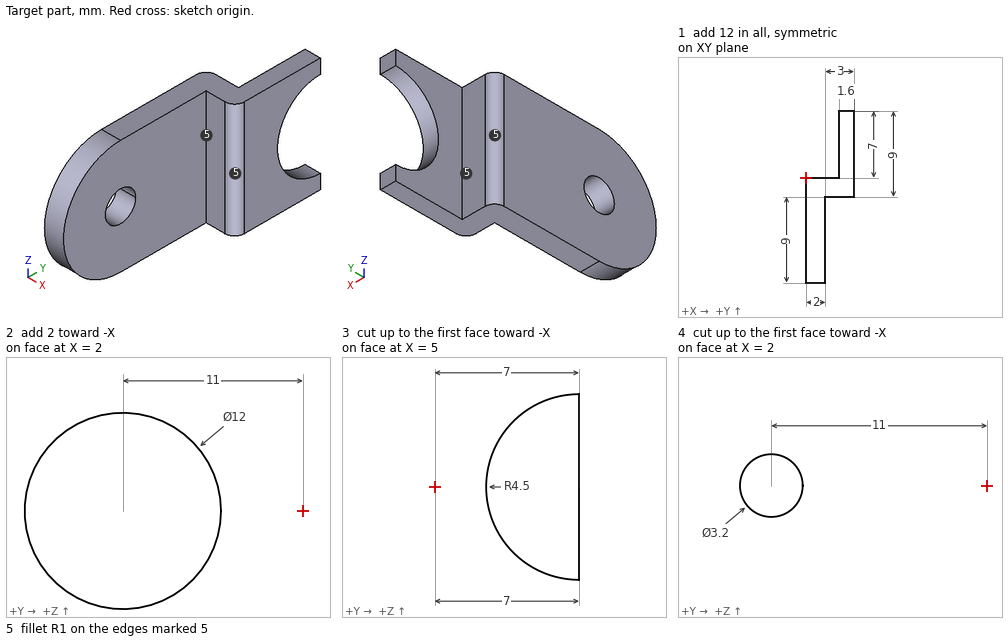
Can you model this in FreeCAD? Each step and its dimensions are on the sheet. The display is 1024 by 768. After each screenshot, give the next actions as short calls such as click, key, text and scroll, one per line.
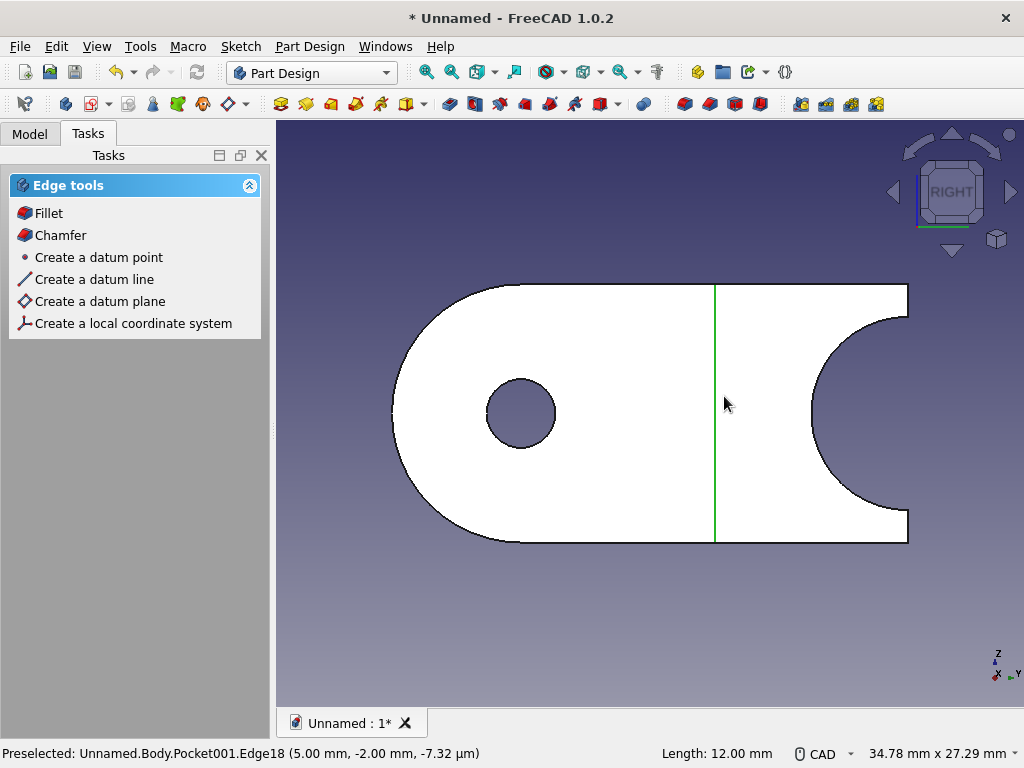
key(5)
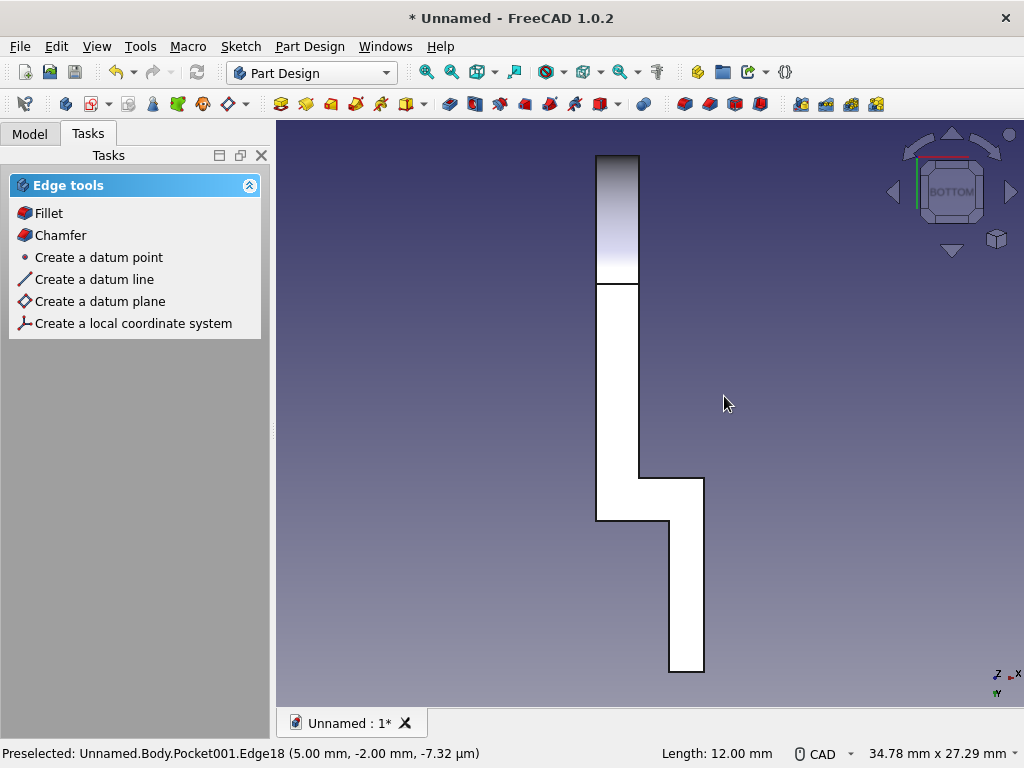
key(4)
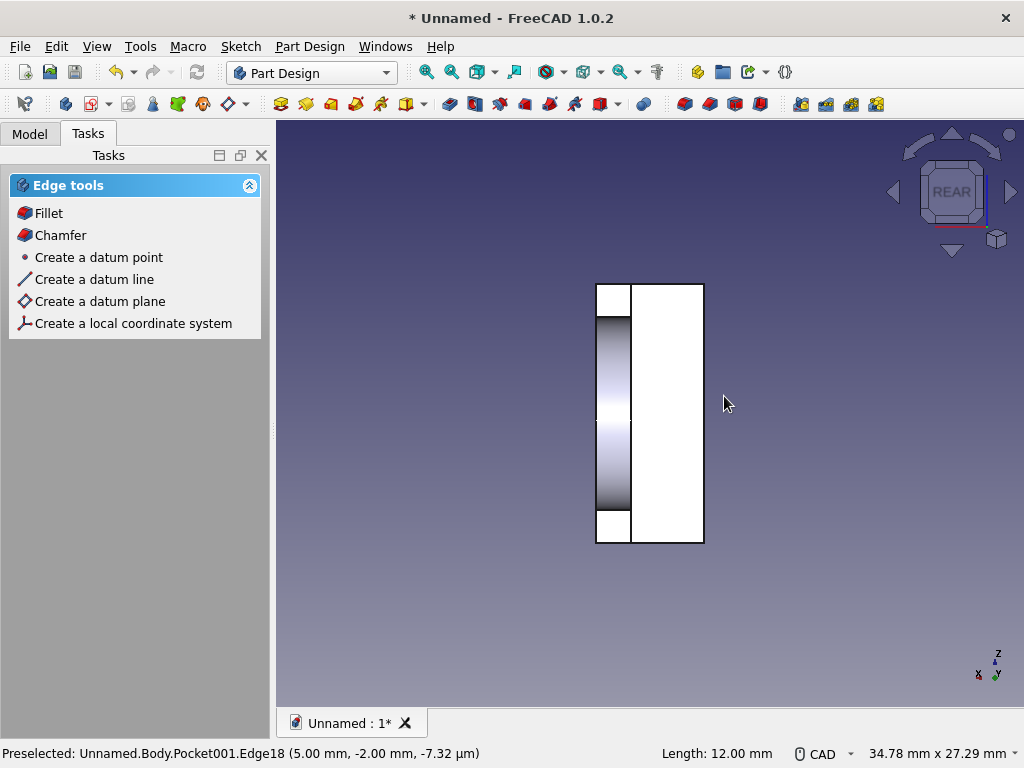
key(v)
key(f)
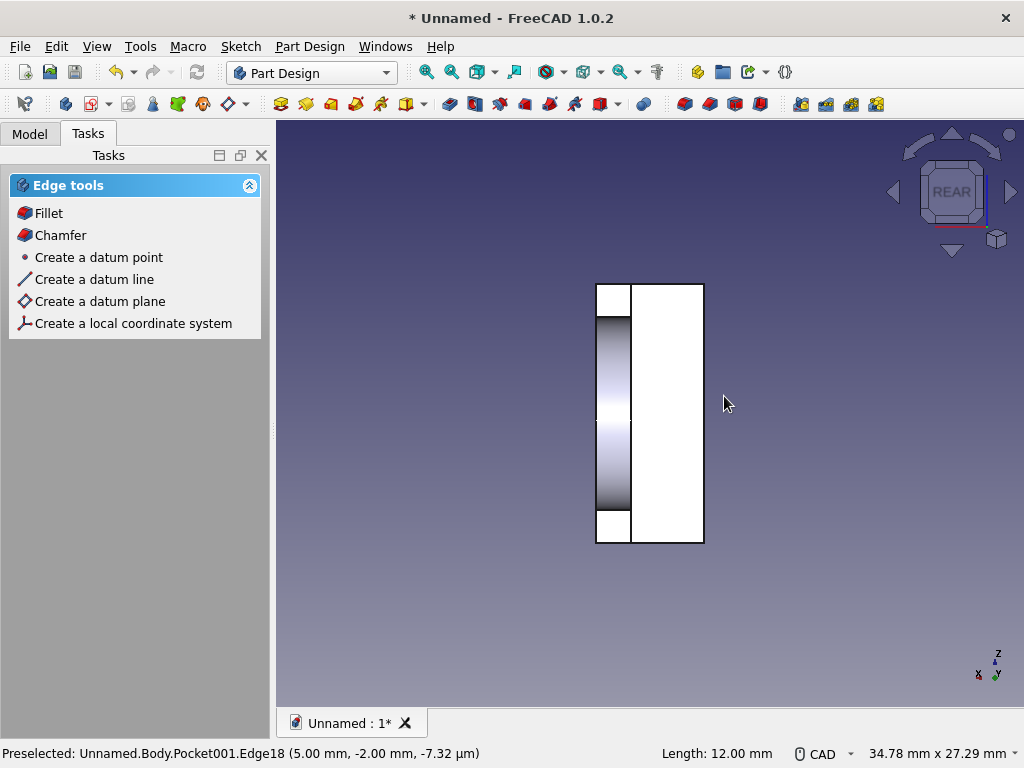
click(704, 413, ctrl)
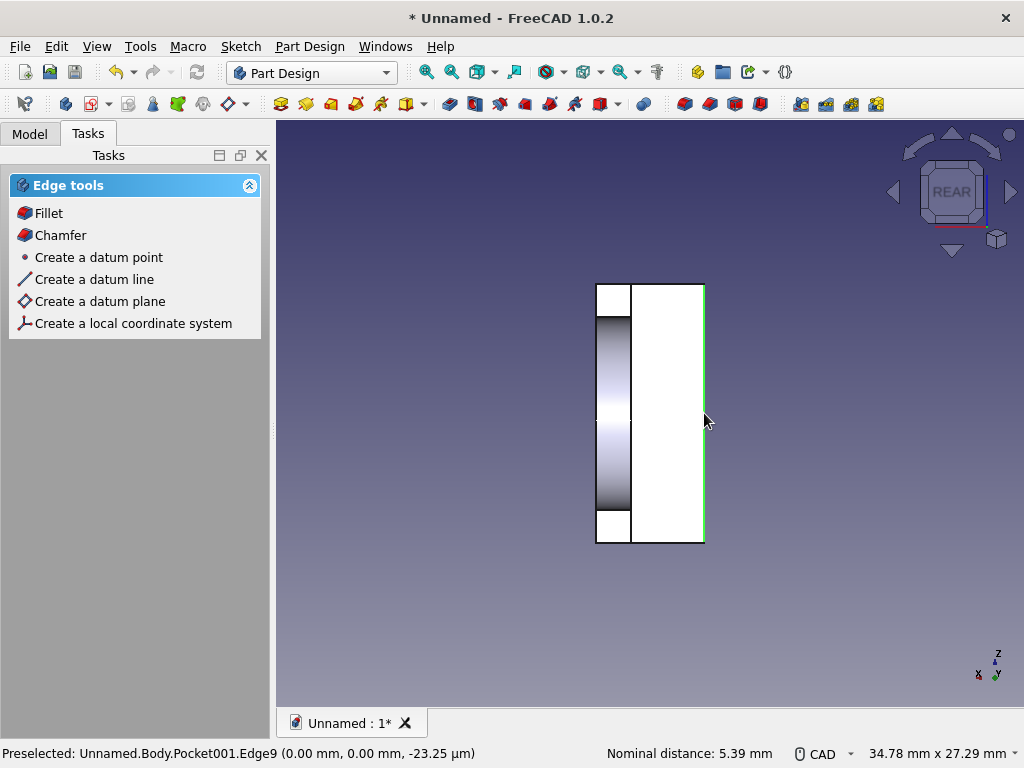
click(685, 104)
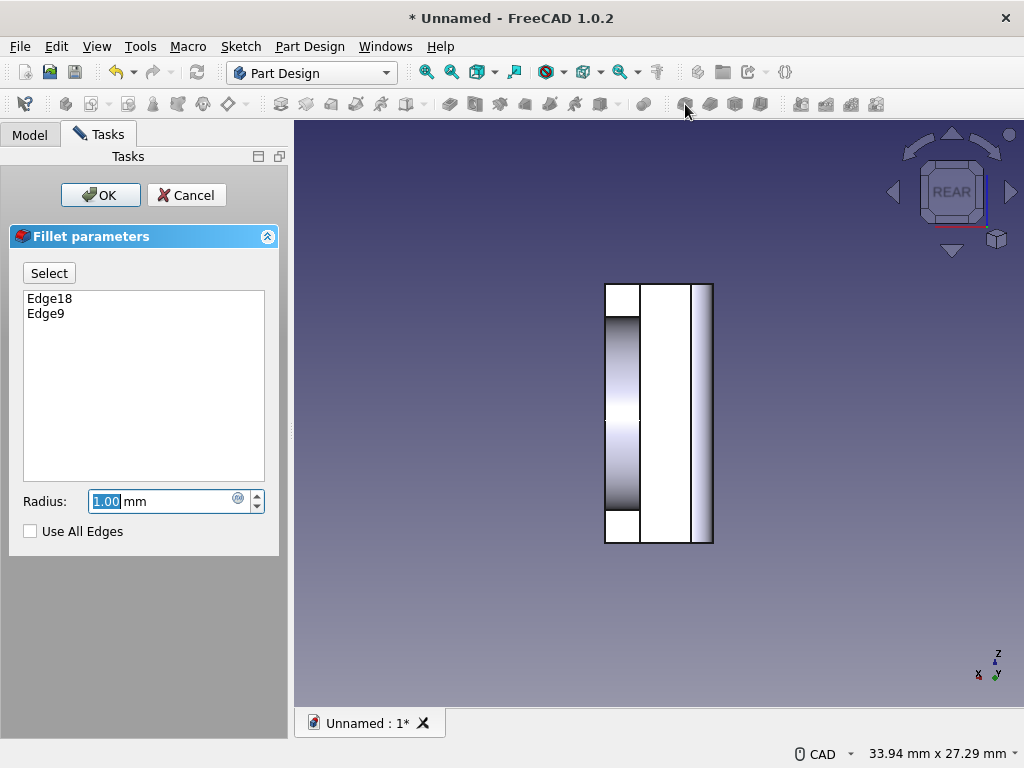
text(1)
key(Tab)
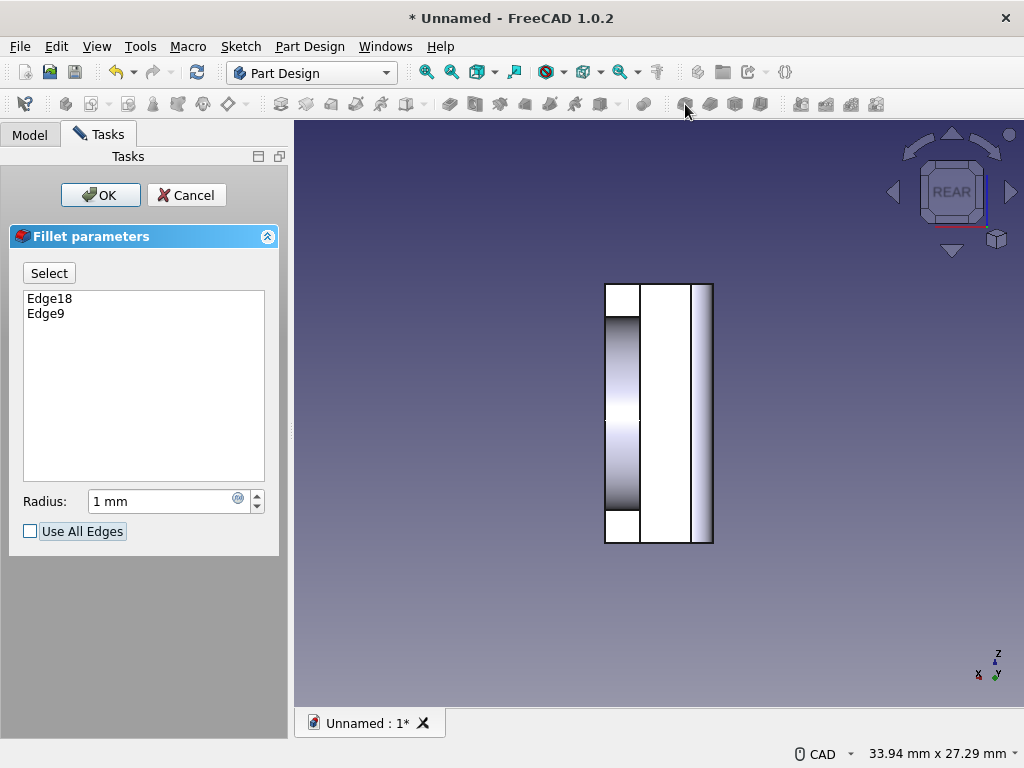
click(101, 195)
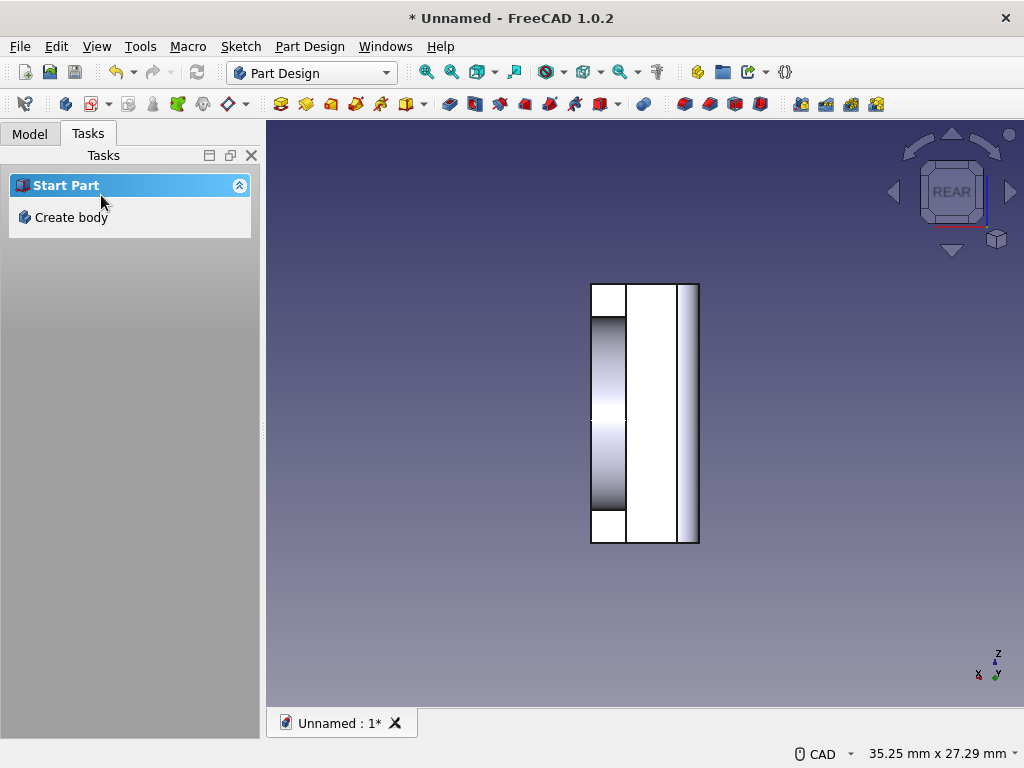
key(0)